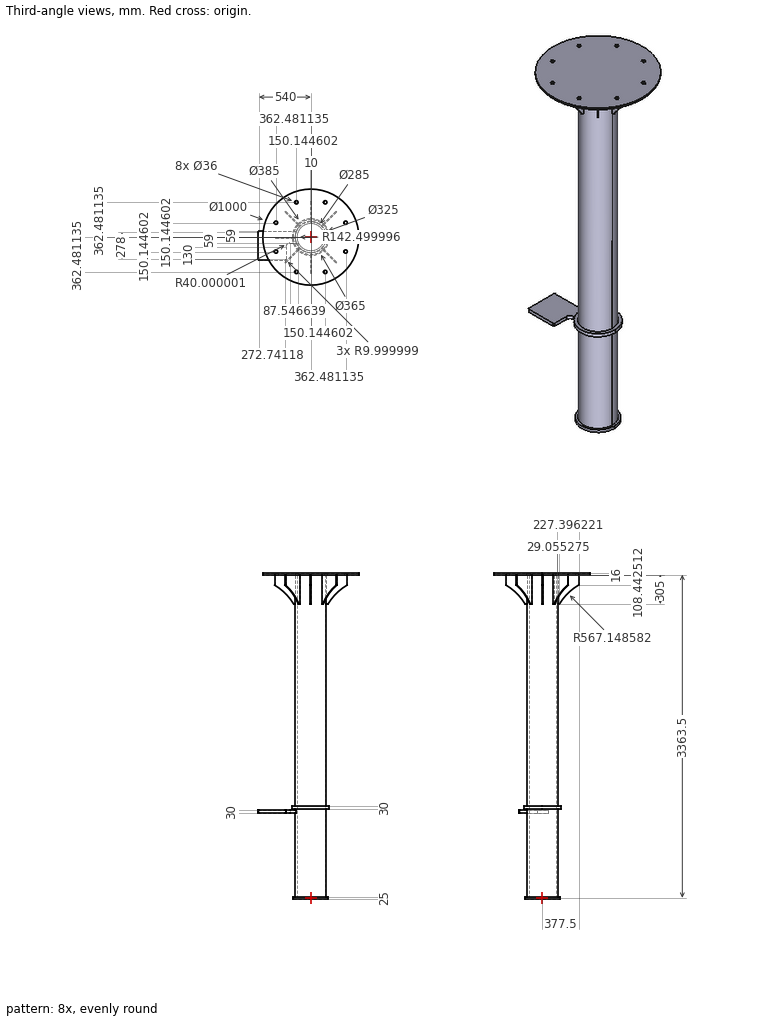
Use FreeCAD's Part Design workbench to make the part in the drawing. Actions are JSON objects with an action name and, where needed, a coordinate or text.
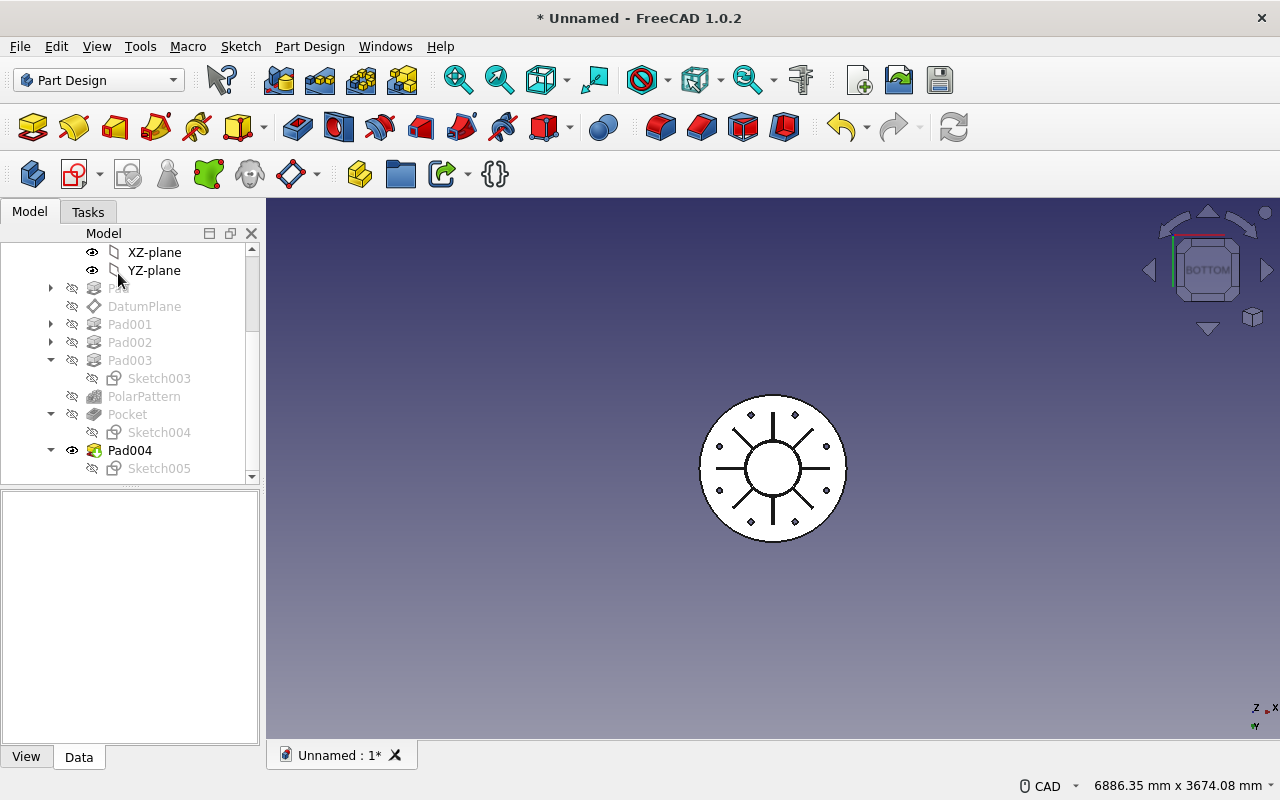
{"action": "scroll", "coordinate": [161, 356], "scroll_direction": "down", "scroll_amount": 3}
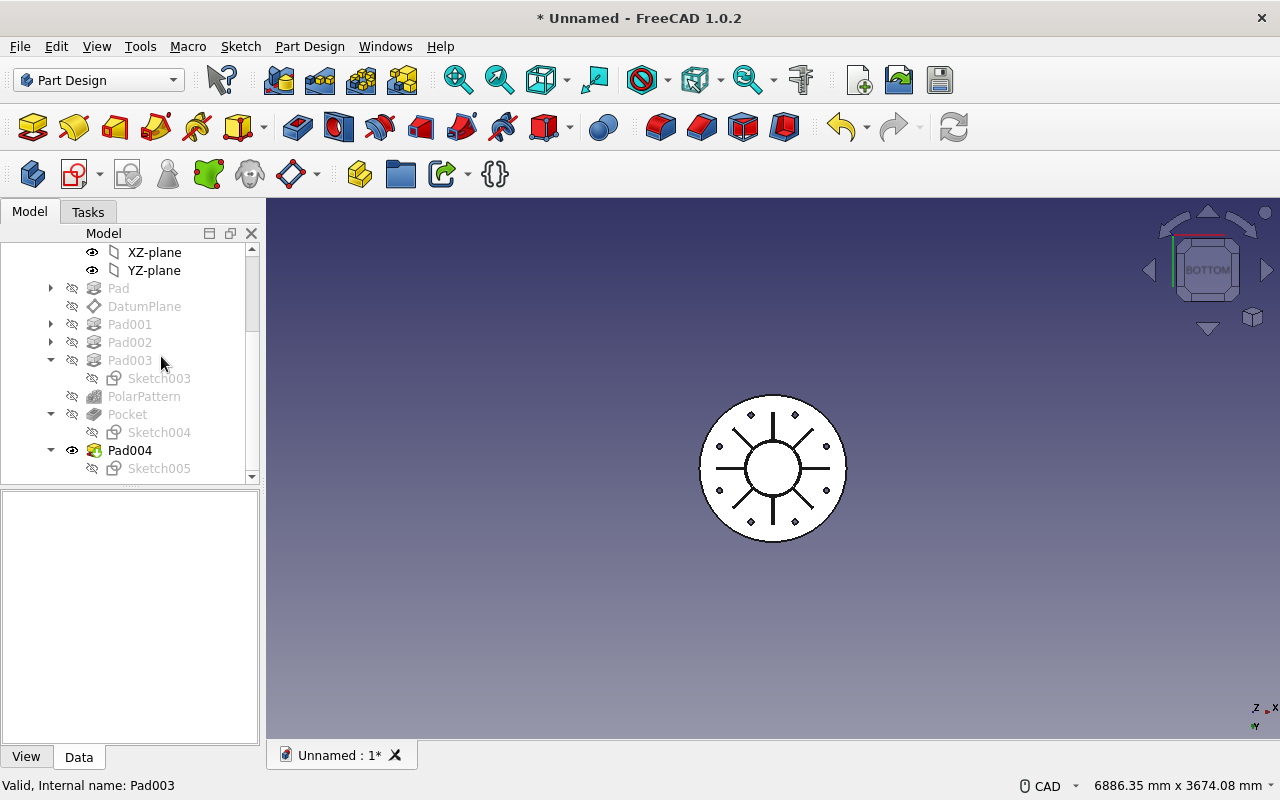
{"action": "scroll", "coordinate": [161, 356], "scroll_direction": "up", "scroll_amount": 15}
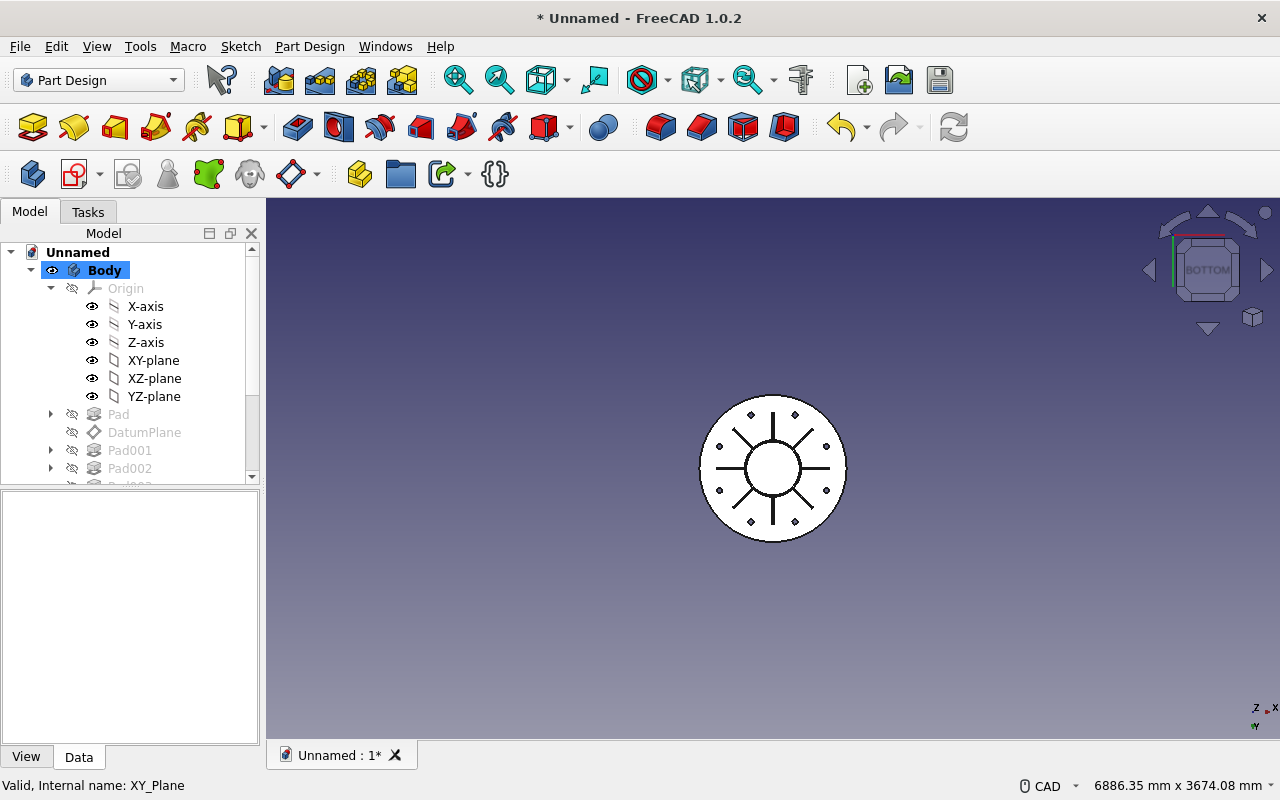
{"action": "left_click", "coordinate": [137, 360]}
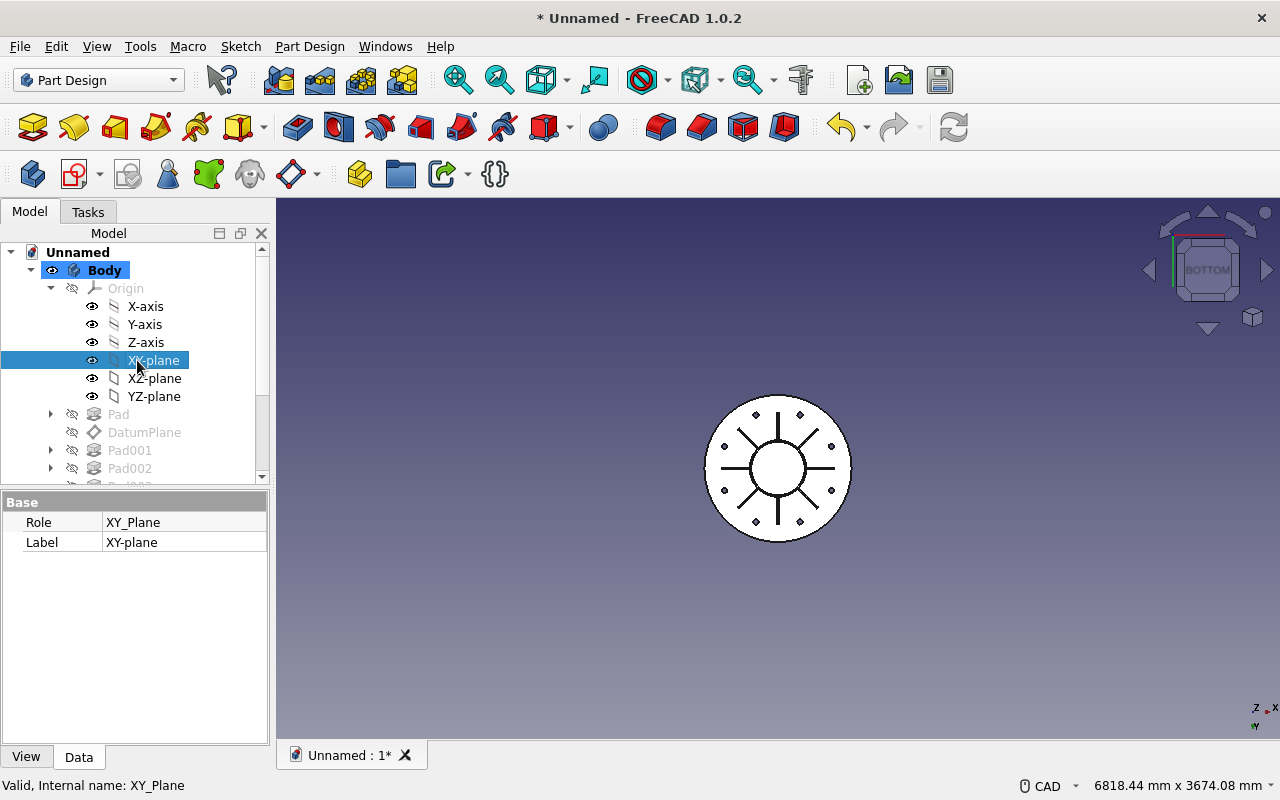
{"action": "left_click", "coordinate": [290, 174]}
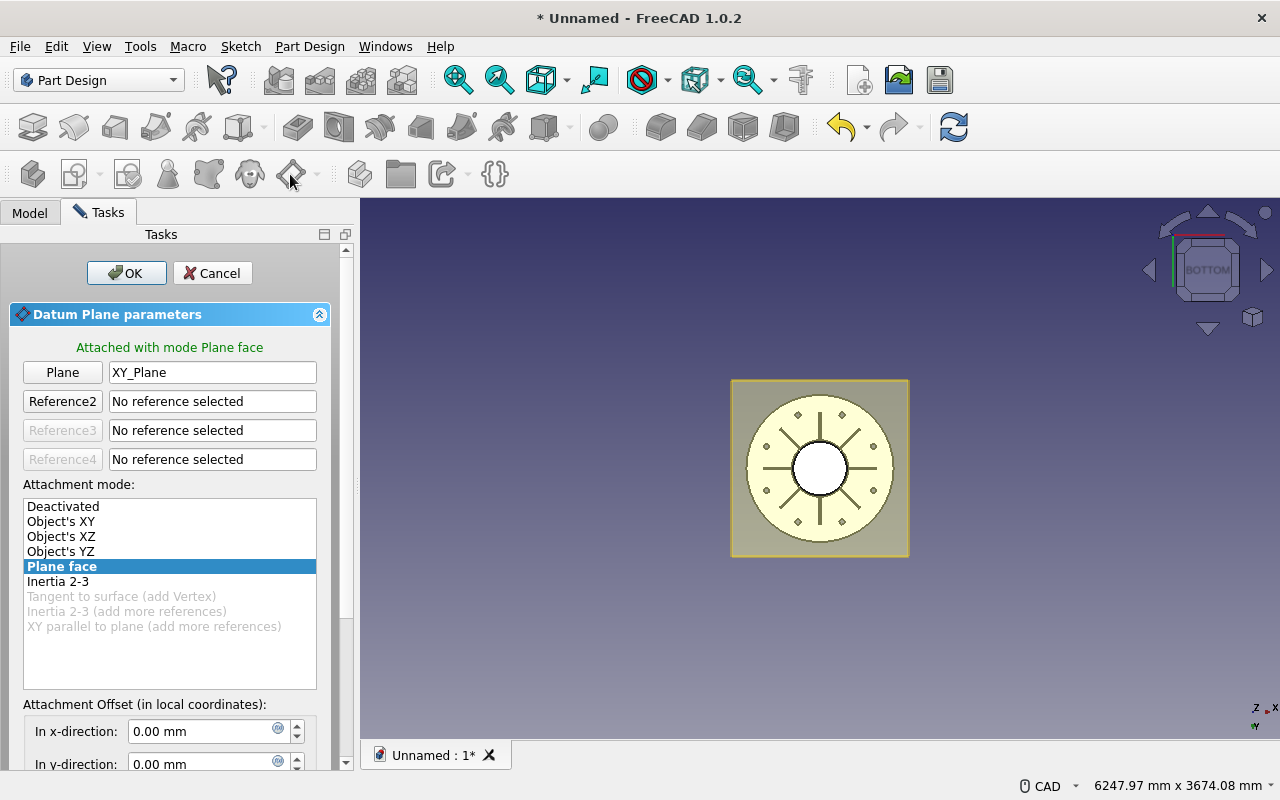
{"action": "scroll", "coordinate": [346, 507], "scroll_direction": "down", "scroll_amount": 2}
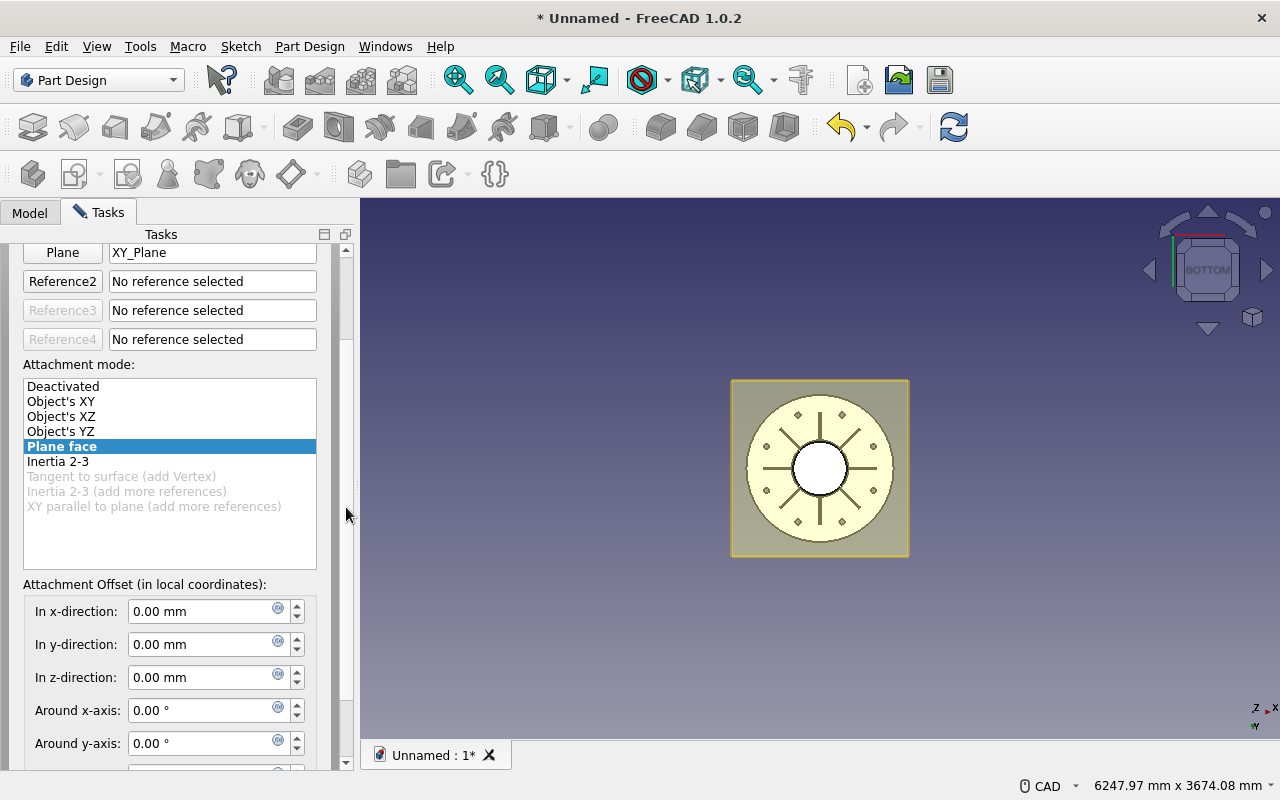
{"action": "triple_click", "coordinate": [210, 678]}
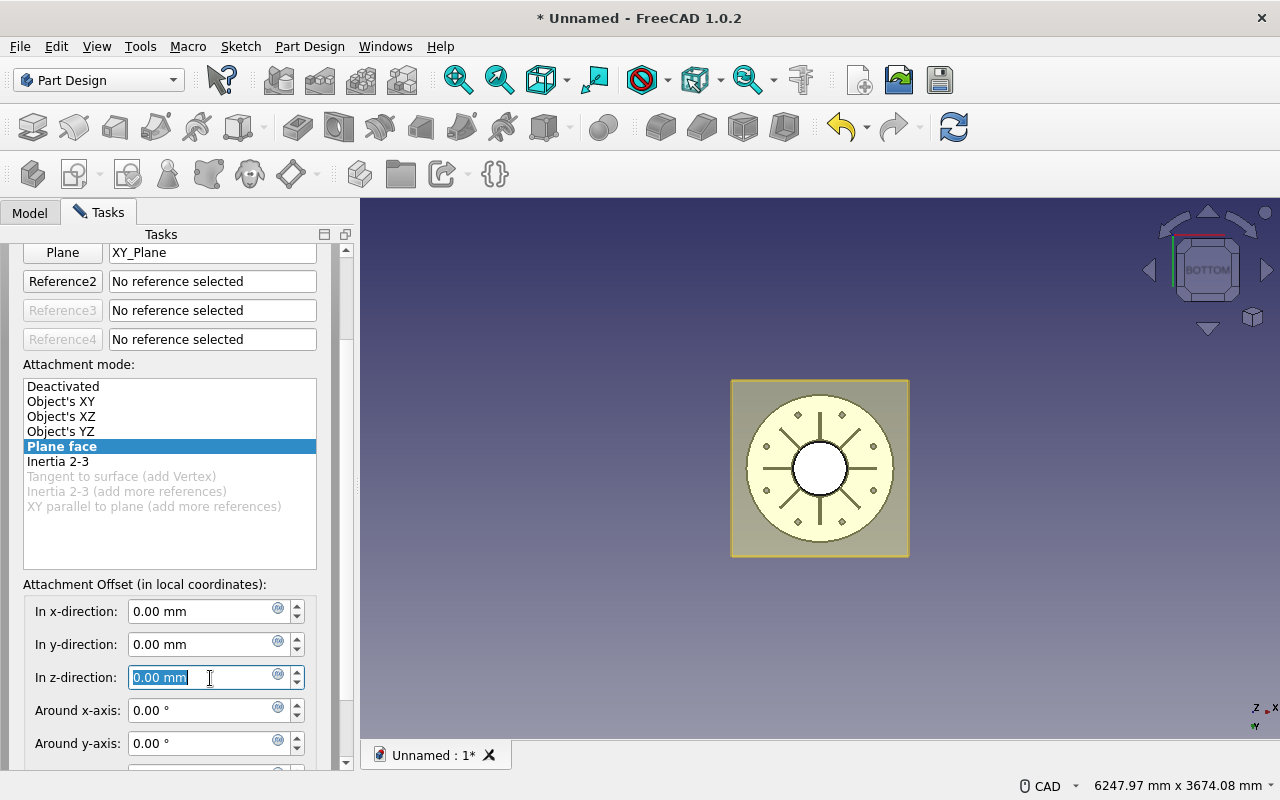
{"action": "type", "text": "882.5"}
{"action": "key", "text": "Tab"}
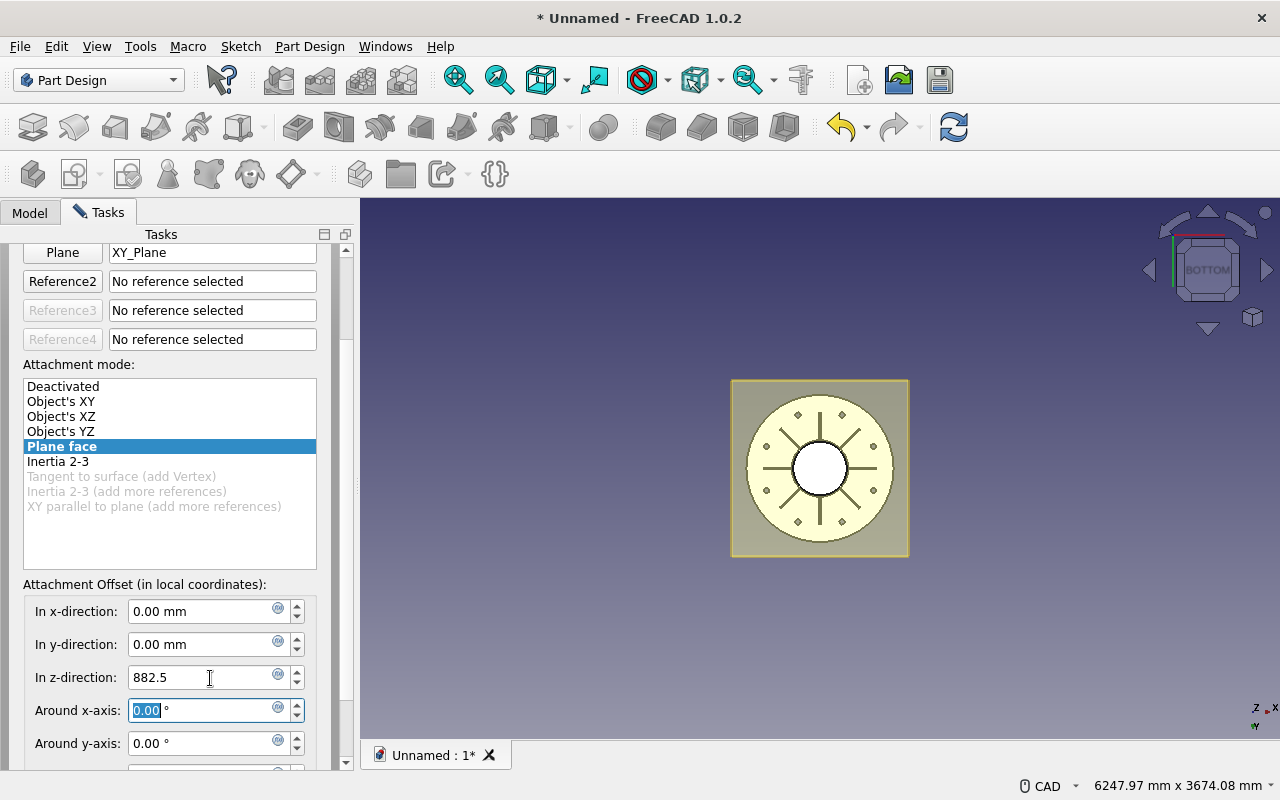
{"action": "scroll", "coordinate": [346, 507], "scroll_direction": "up", "scroll_amount": 3}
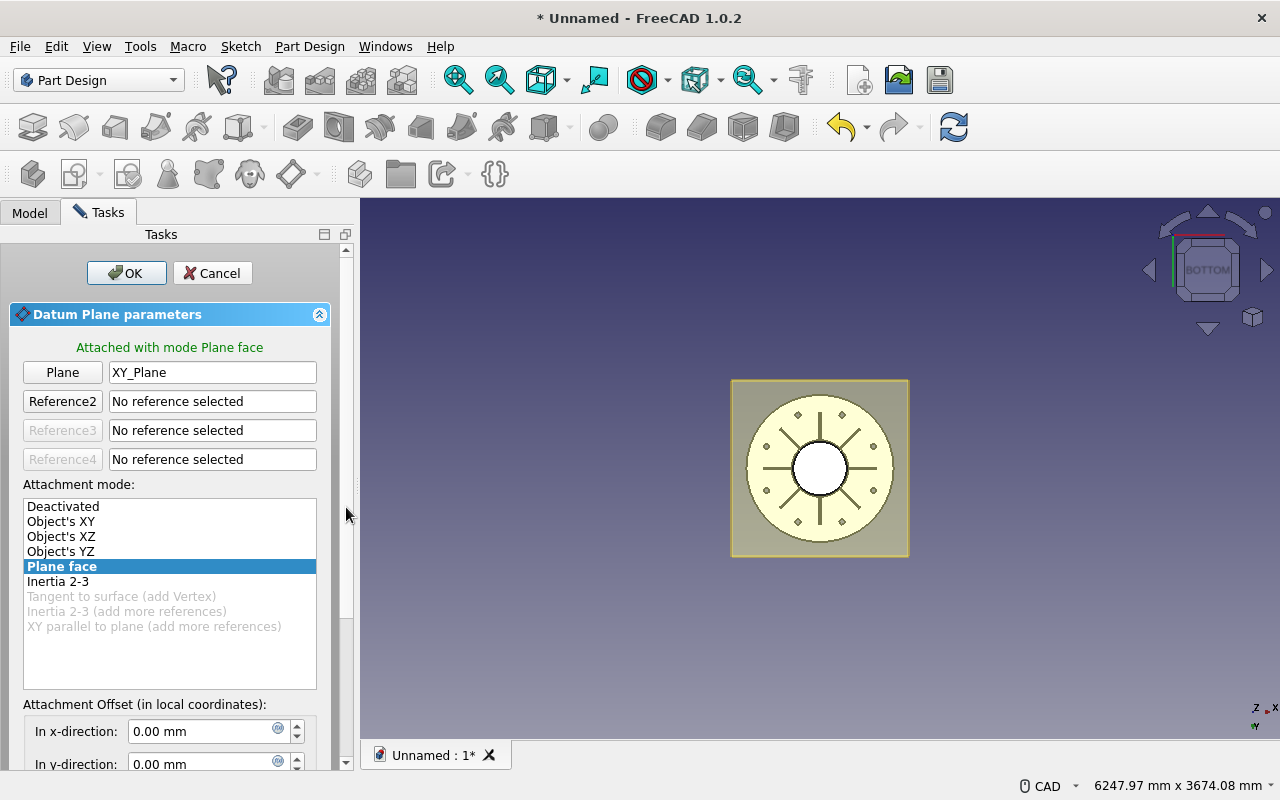
{"action": "left_click", "coordinate": [127, 273]}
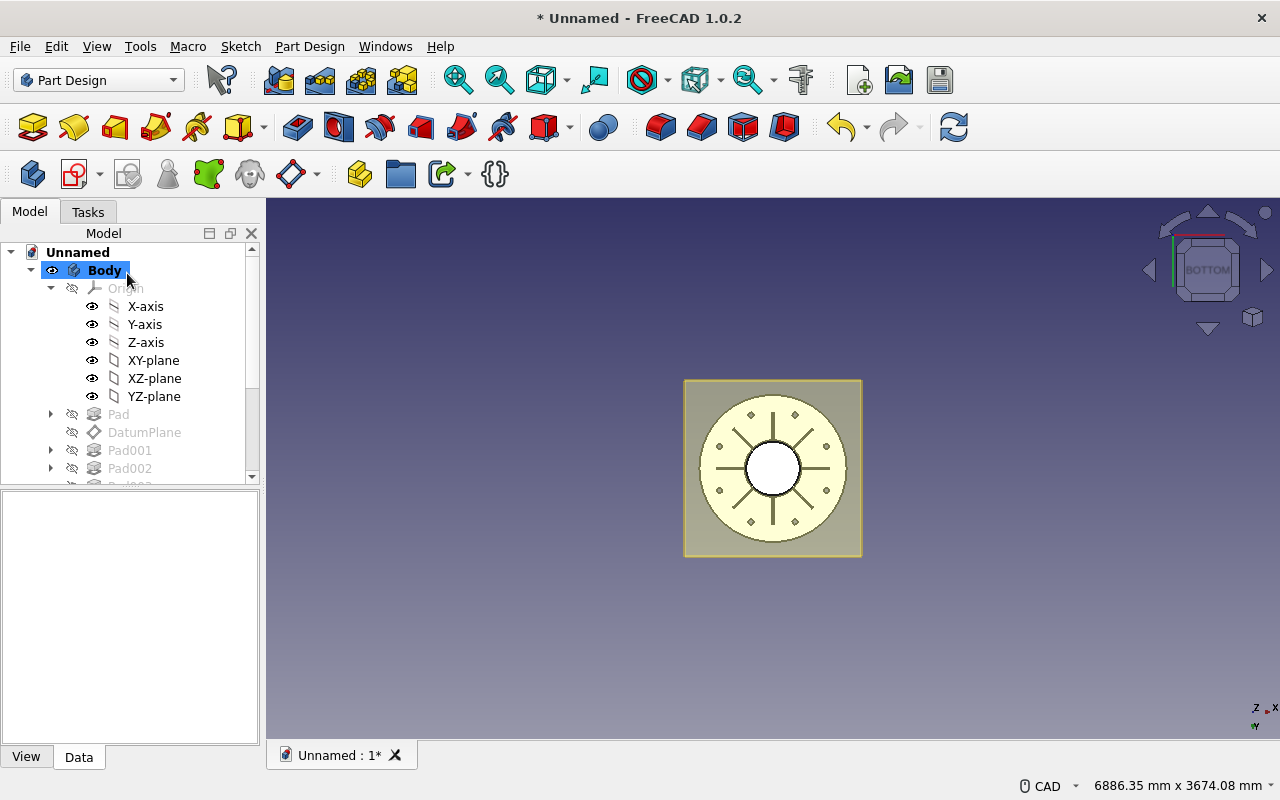
{"action": "scroll", "coordinate": [101, 356], "scroll_direction": "down", "scroll_amount": 3}